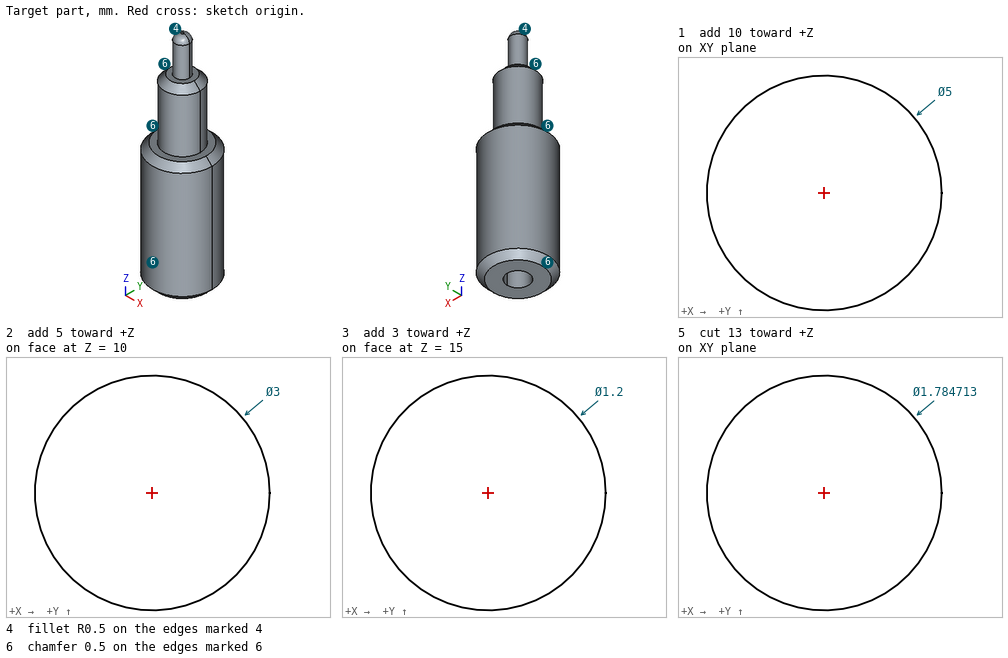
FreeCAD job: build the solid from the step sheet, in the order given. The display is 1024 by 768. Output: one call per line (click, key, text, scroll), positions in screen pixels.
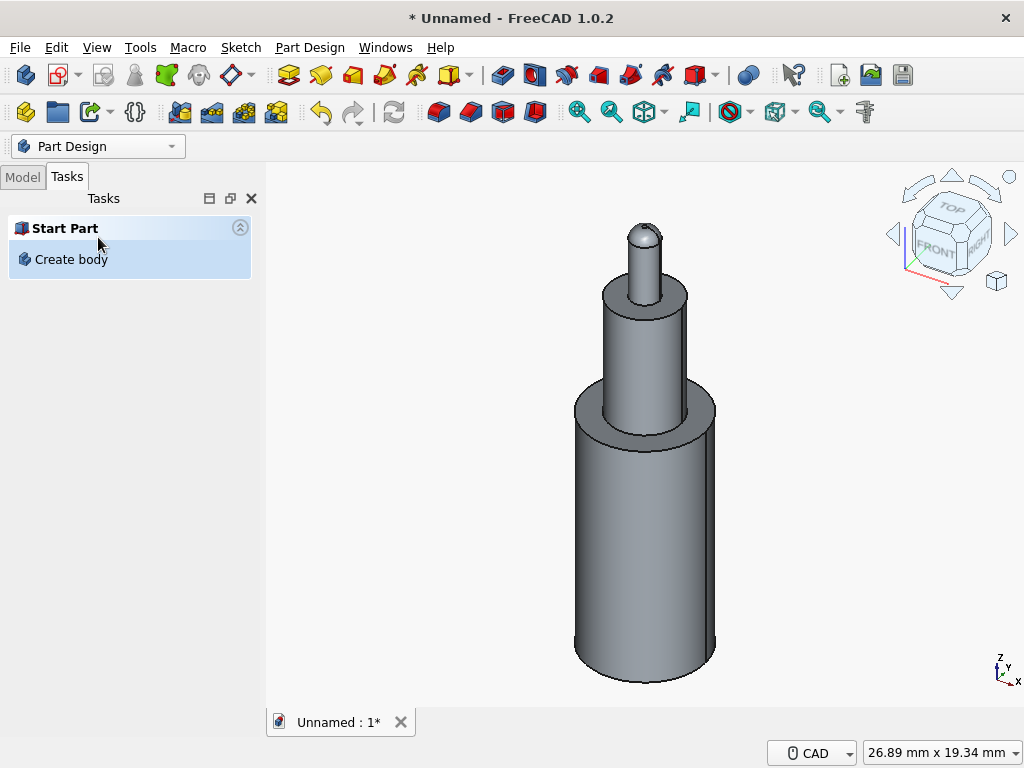
click(58, 76)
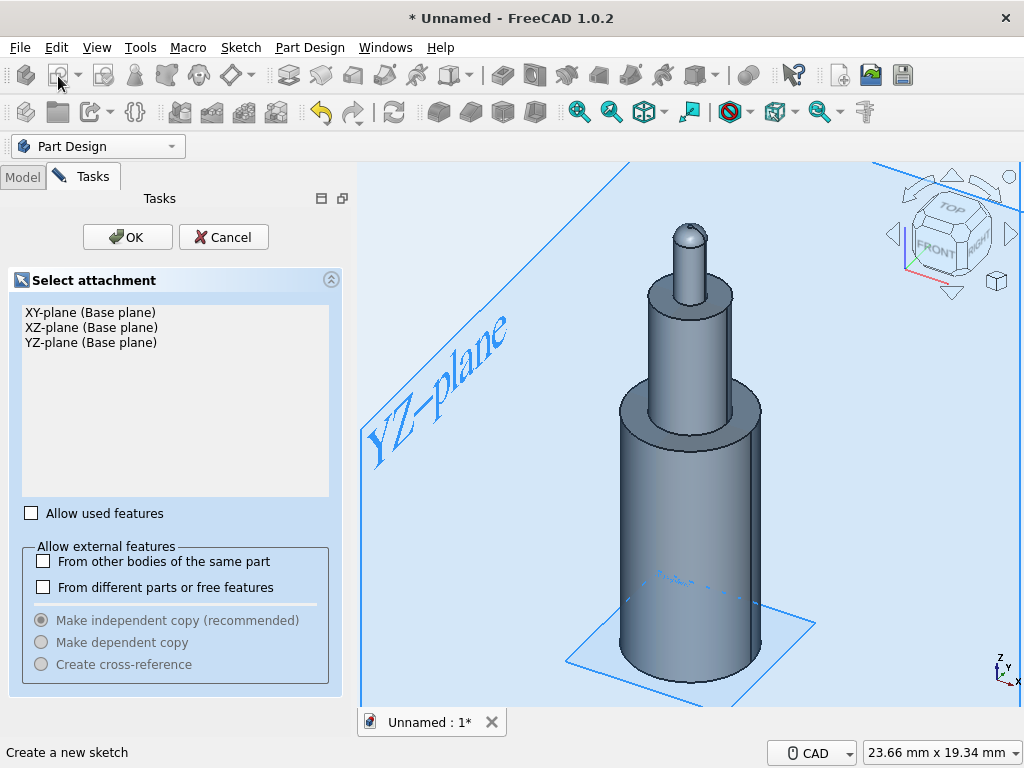
click(82, 312)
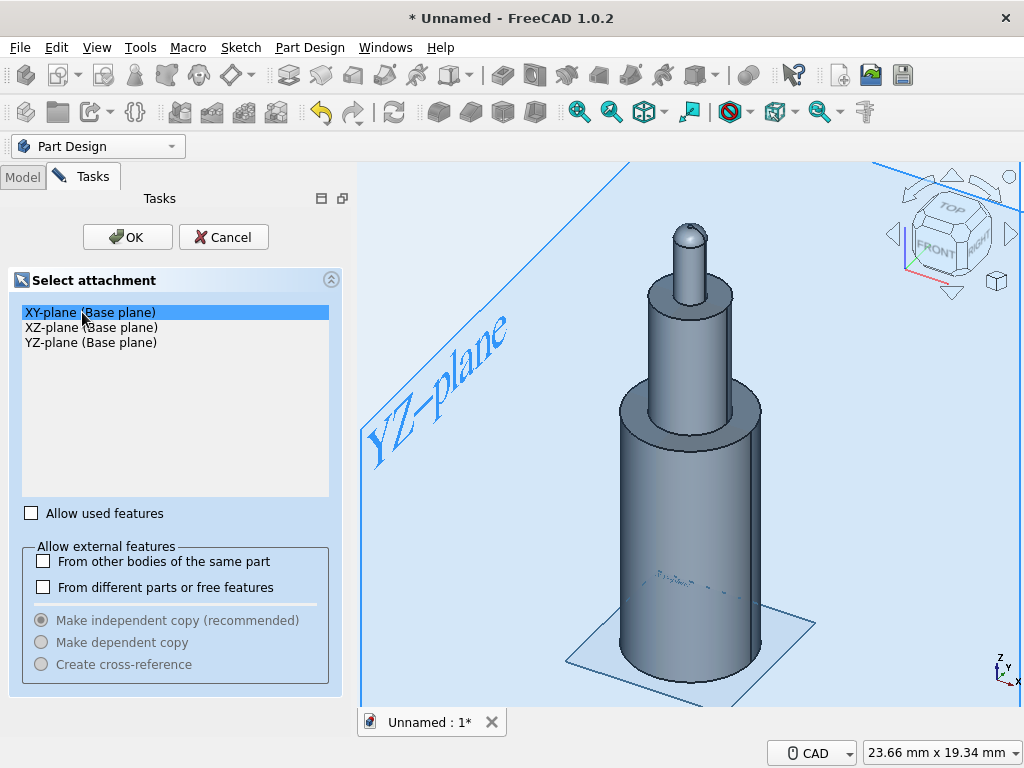
click(128, 237)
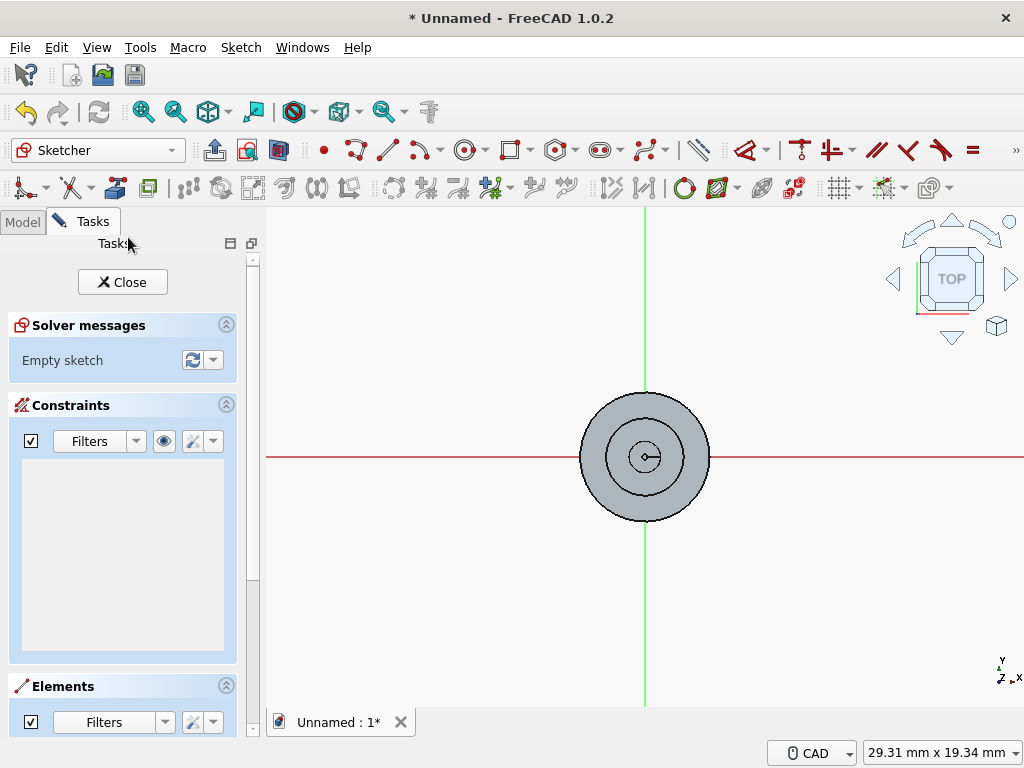
click(280, 150)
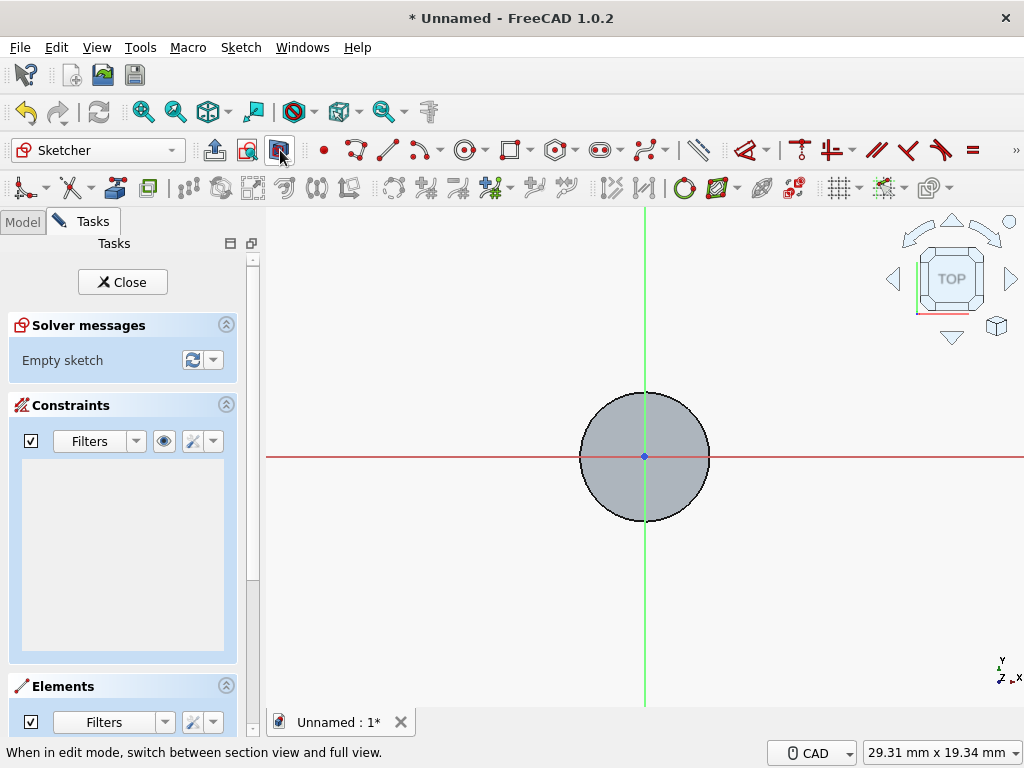
scroll(656, 457, up, 10)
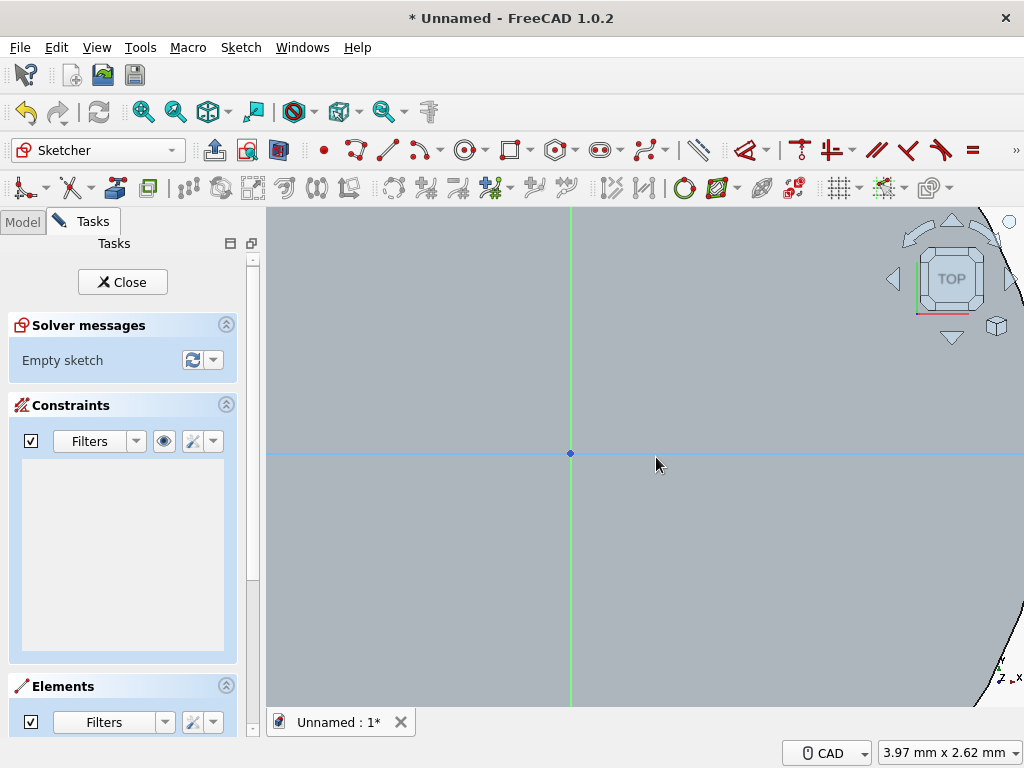
click(466, 150)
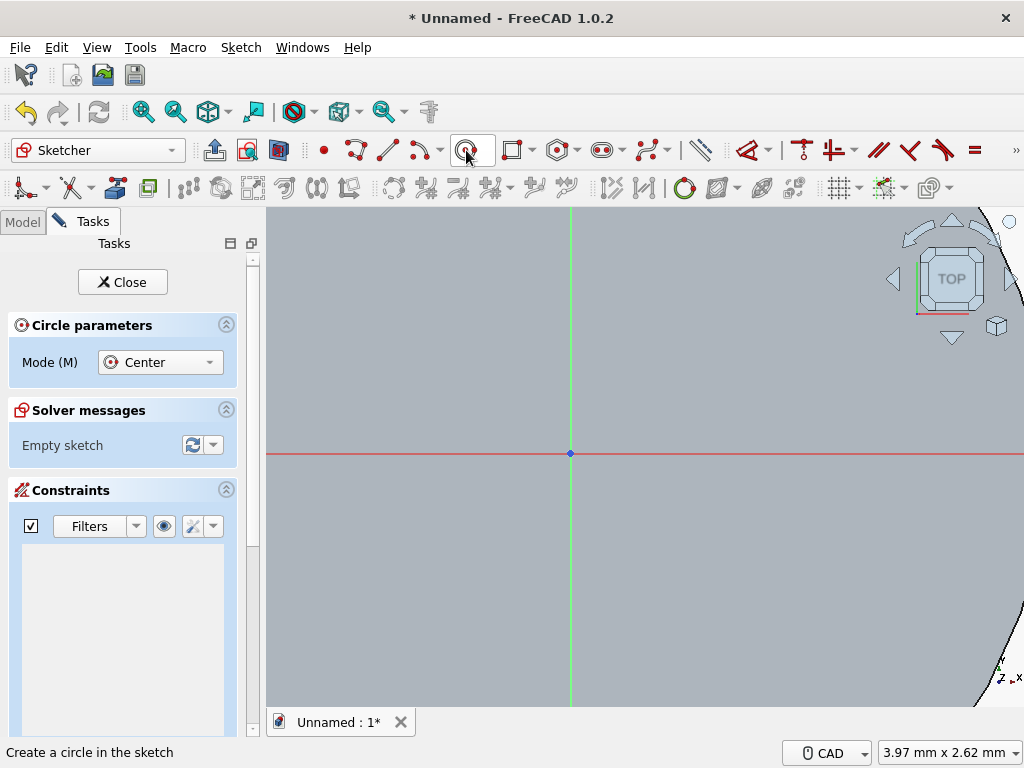
click(571, 454)
move(691, 333)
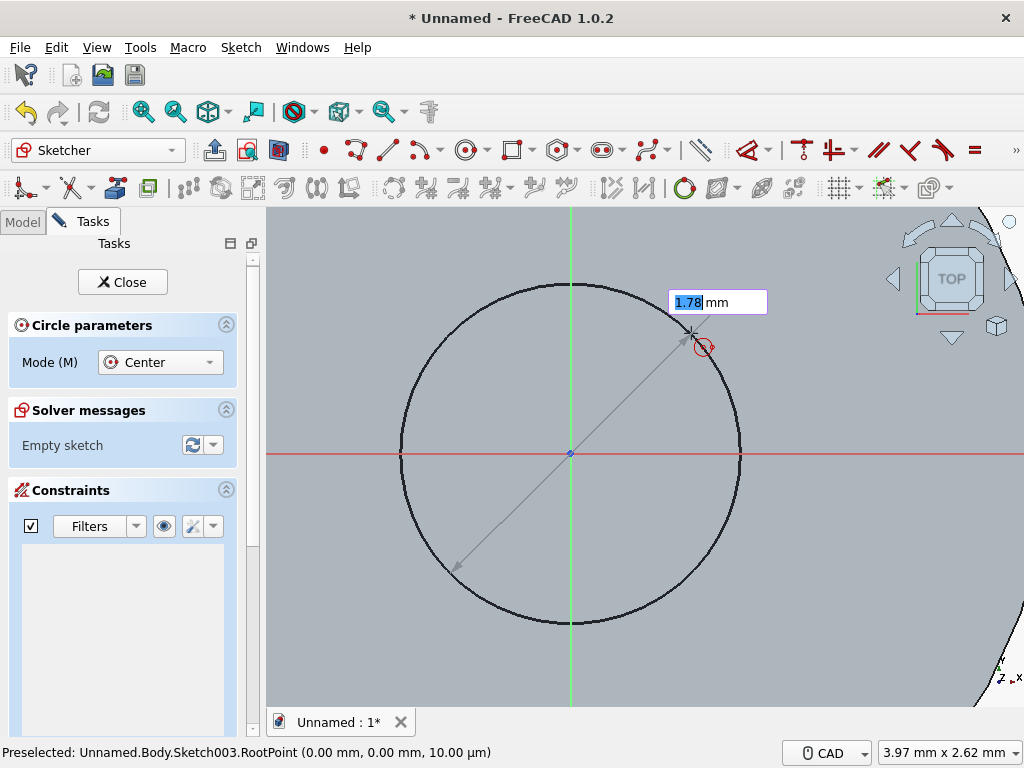
text(1.784713)
key(Return)
key(Escape)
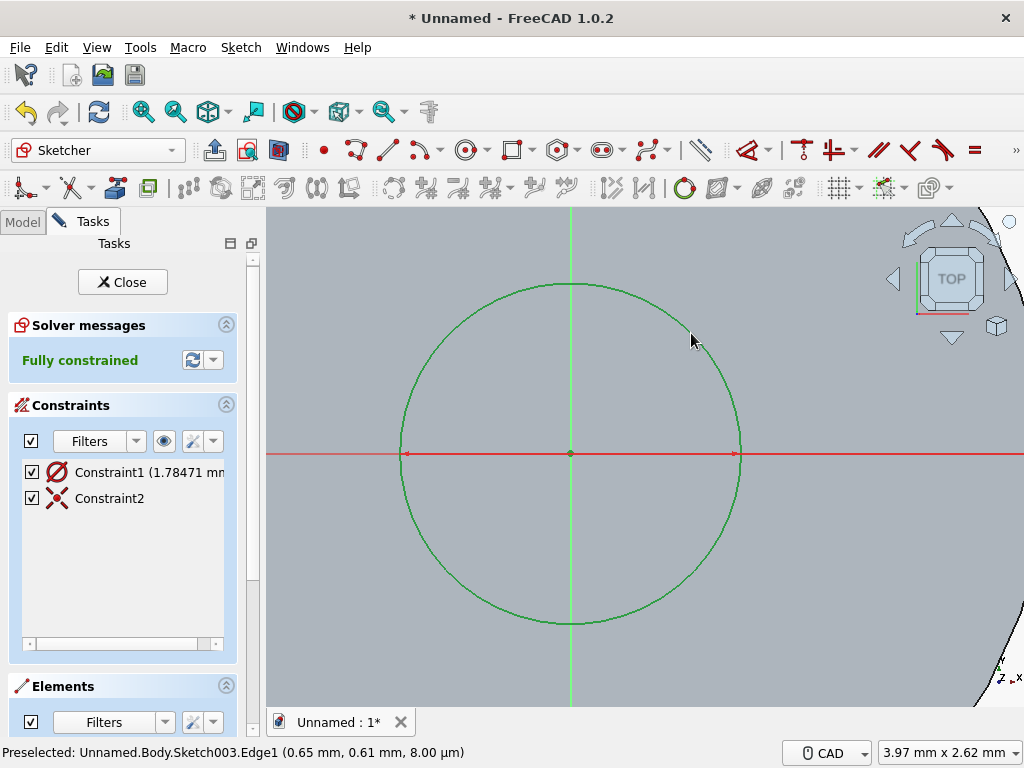
click(123, 282)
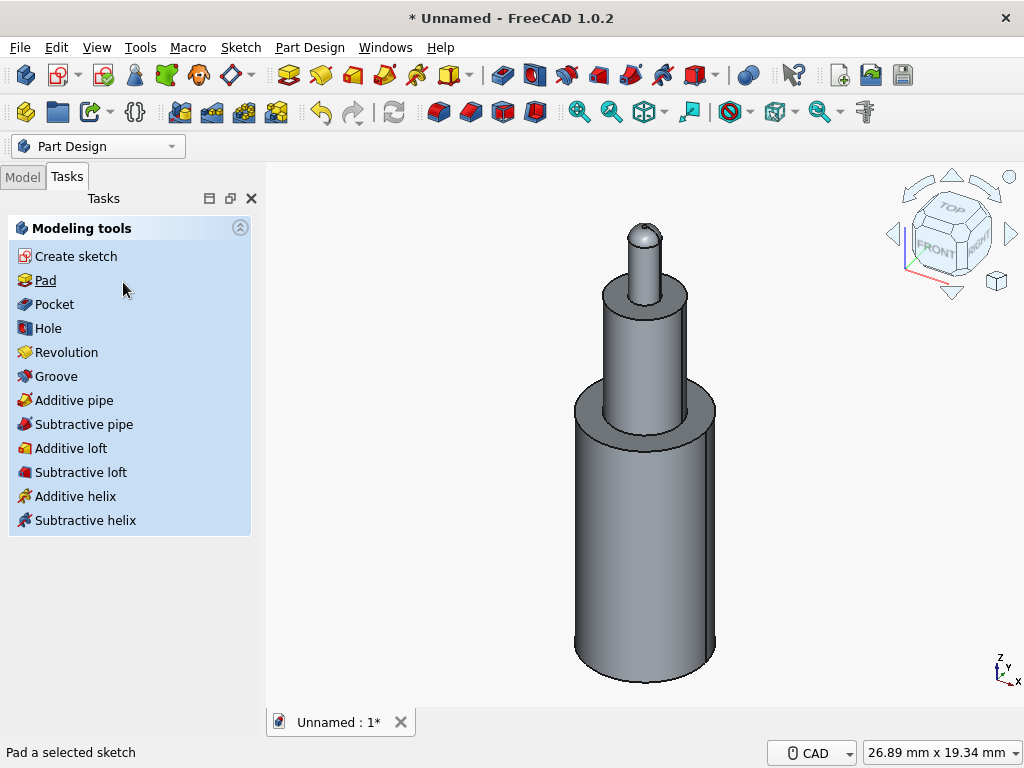
click(504, 76)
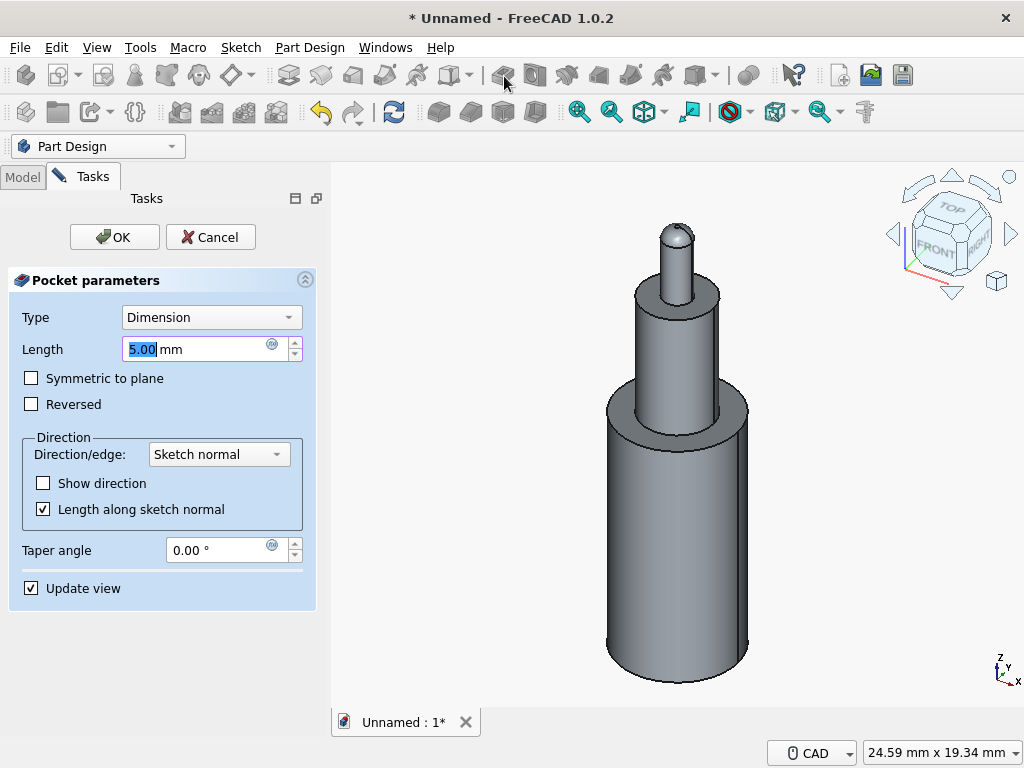
text(13)
key(Tab)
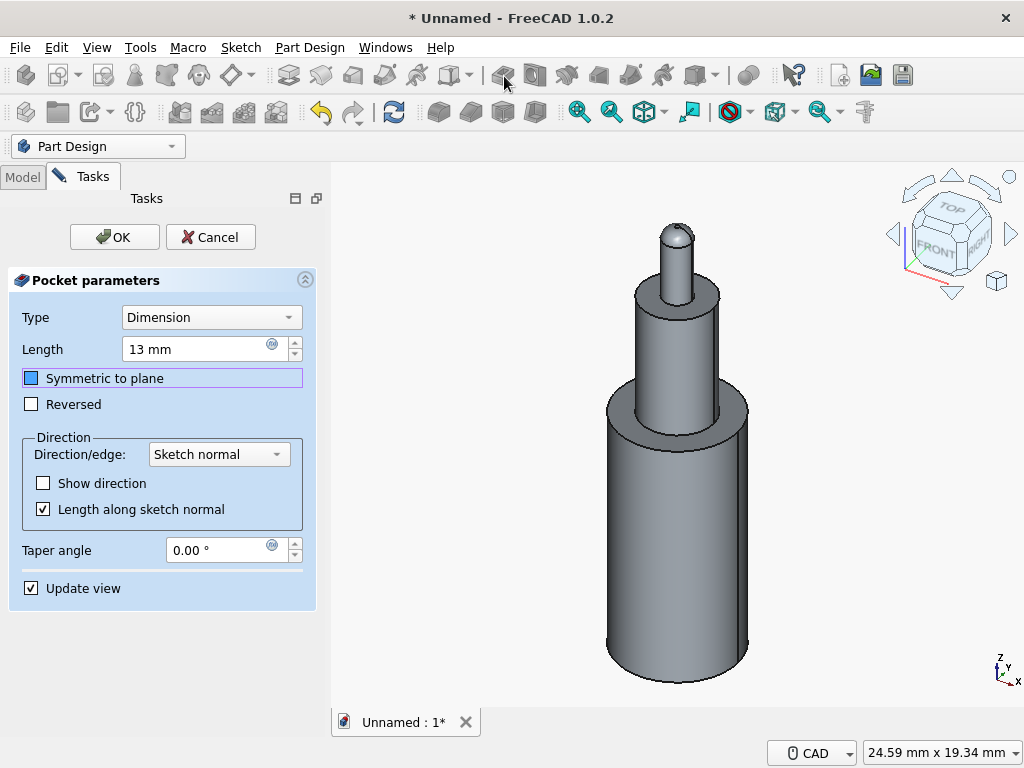
click(30, 404)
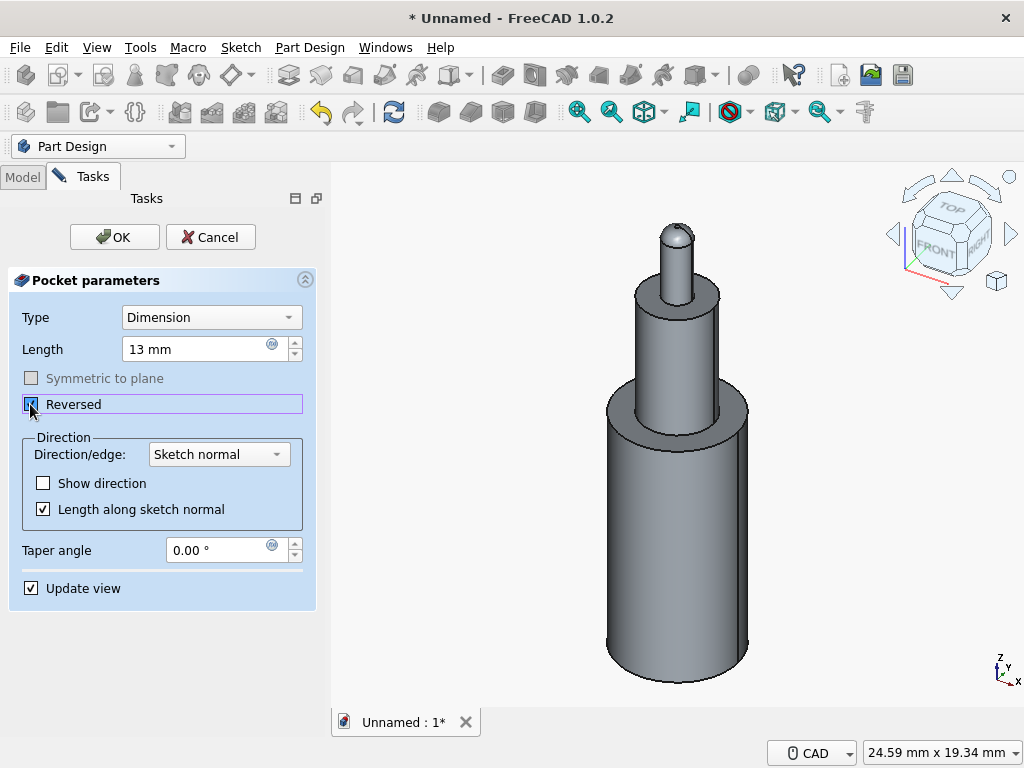
click(115, 237)